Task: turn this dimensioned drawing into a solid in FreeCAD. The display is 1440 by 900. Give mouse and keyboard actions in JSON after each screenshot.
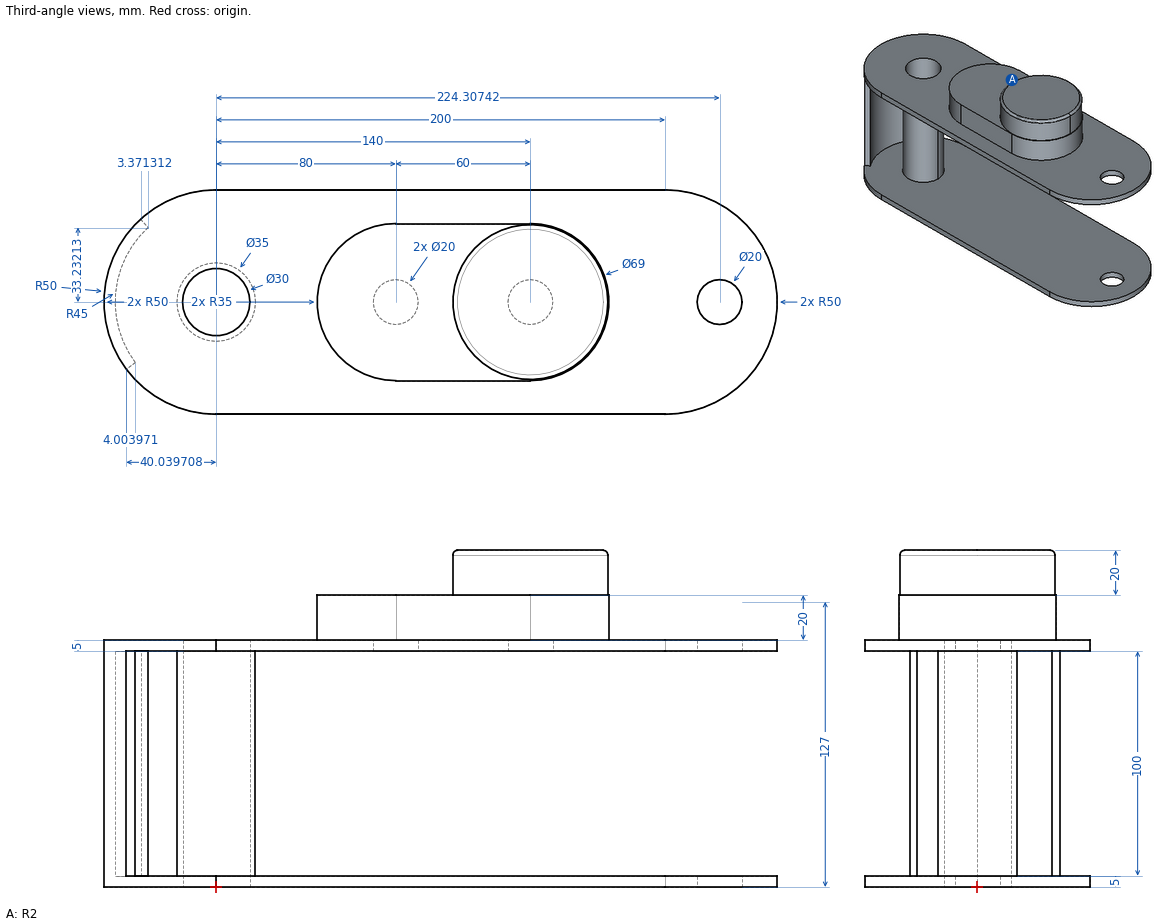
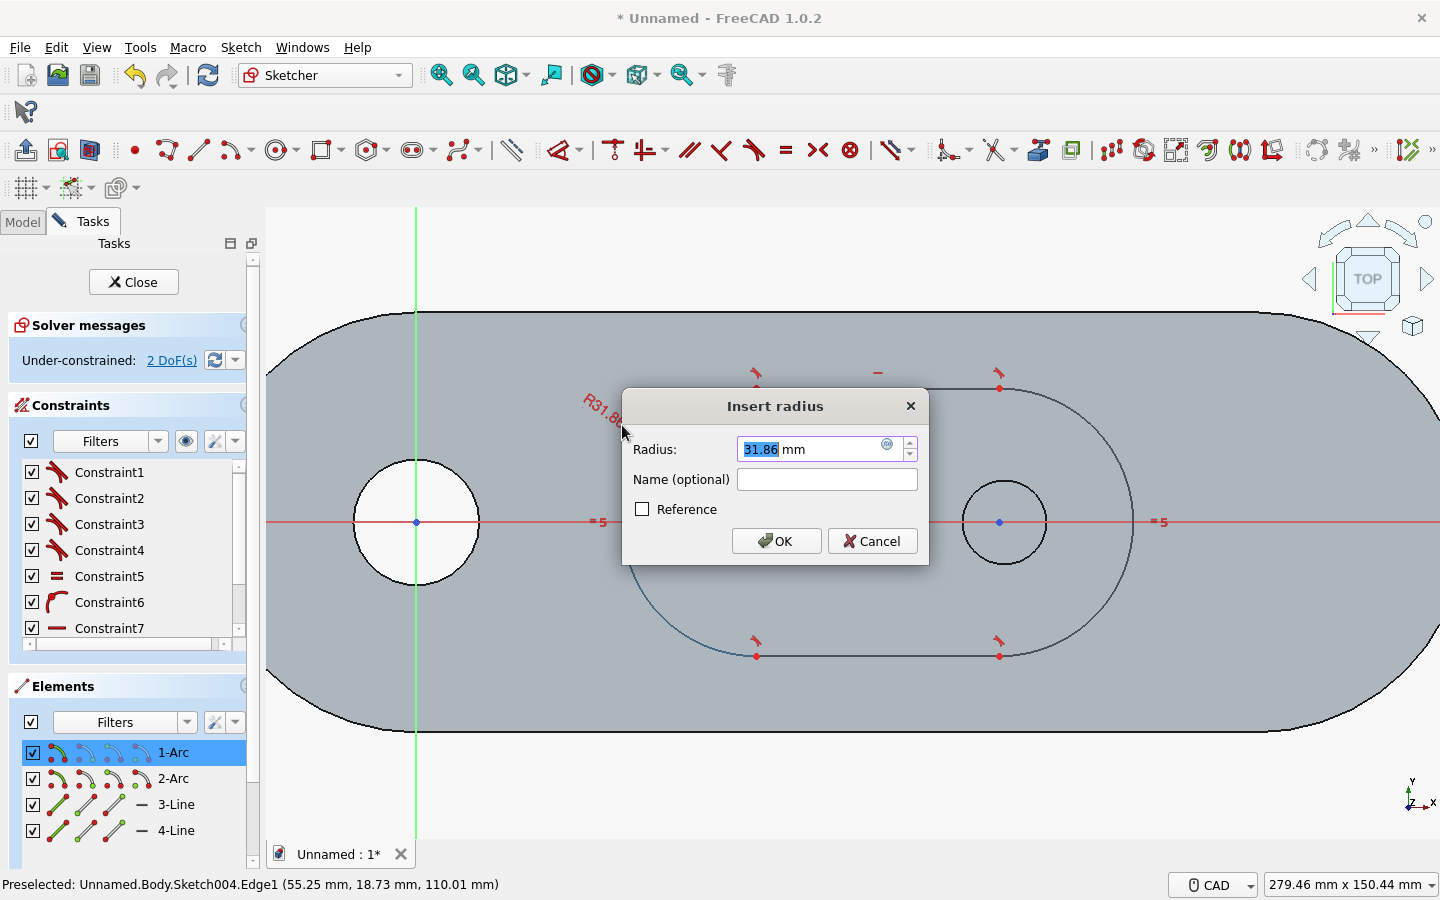
{"action": "type", "text": "35"}
{"action": "key", "text": "Return"}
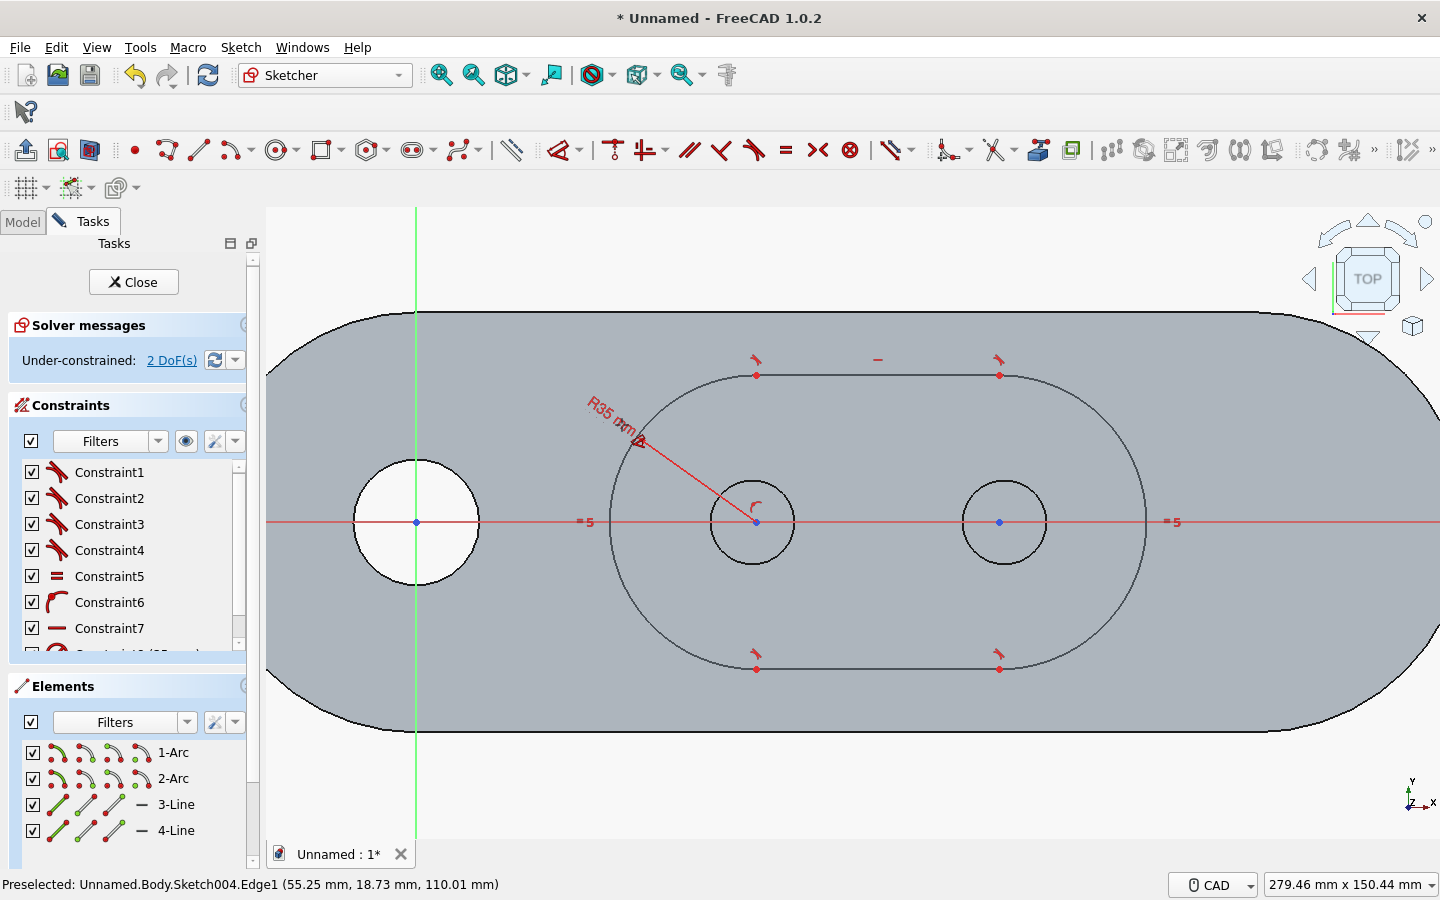
{"action": "left_click", "coordinate": [830, 375]}
{"action": "left_click", "coordinate": [878, 341]}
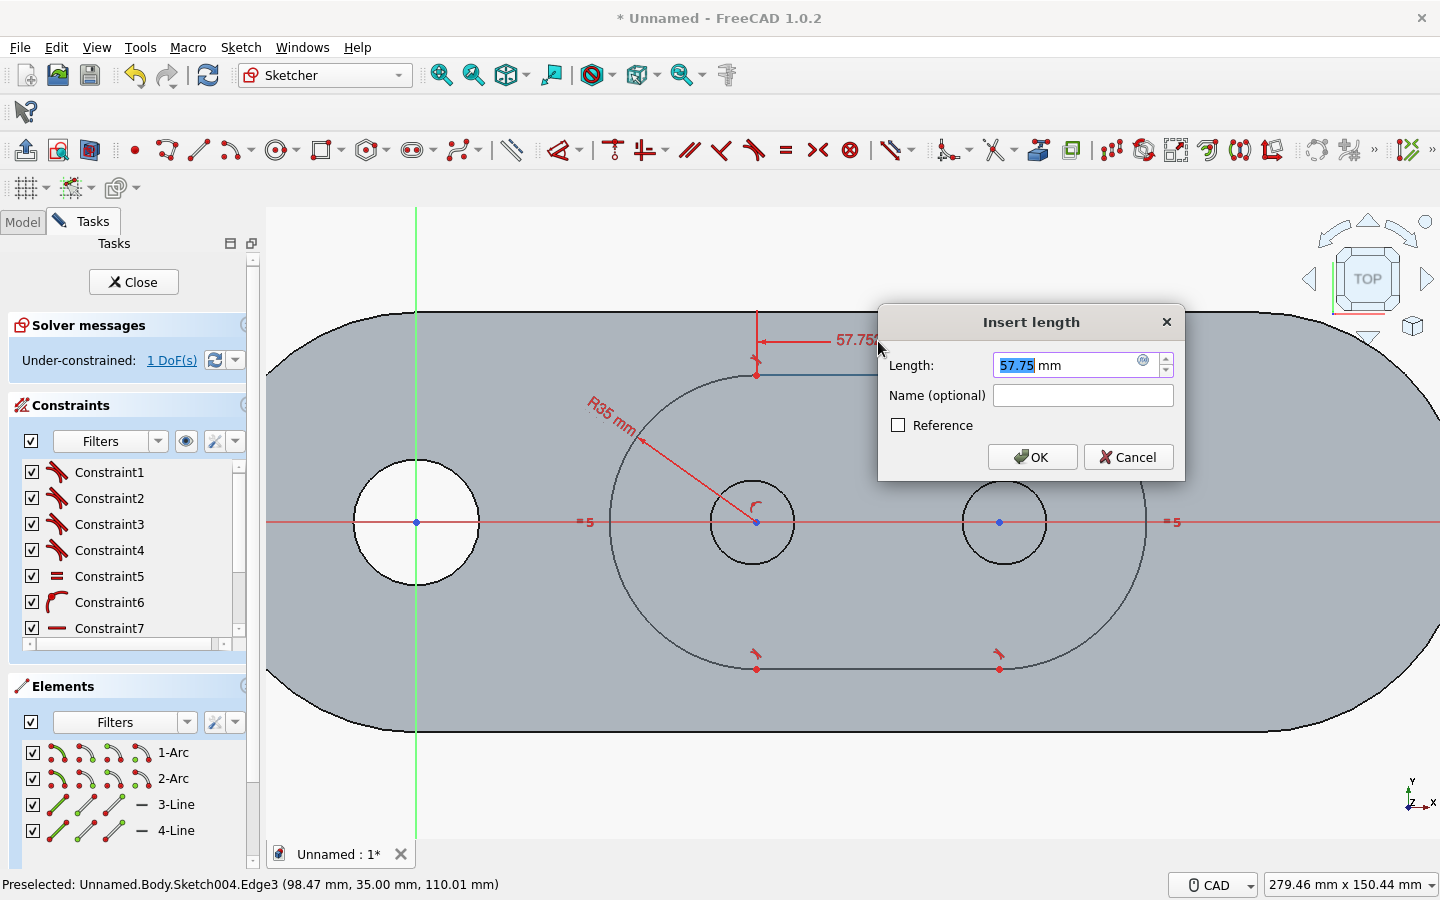
{"action": "type", "text": "60"}
{"action": "key", "text": "Return"}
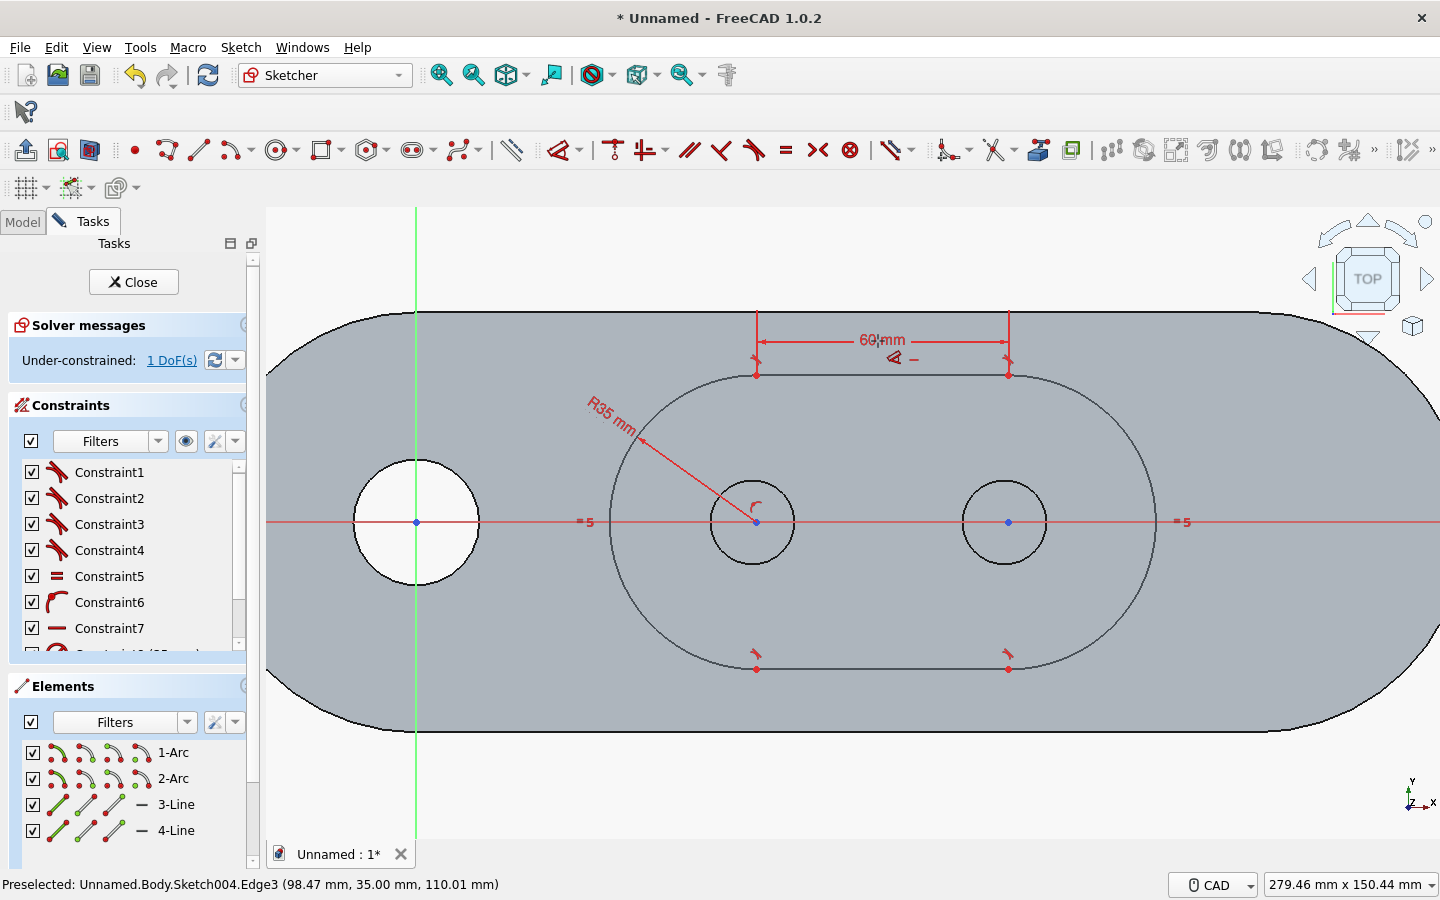
{"action": "left_click", "coordinate": [757, 375]}
{"action": "left_click", "coordinate": [587, 341]}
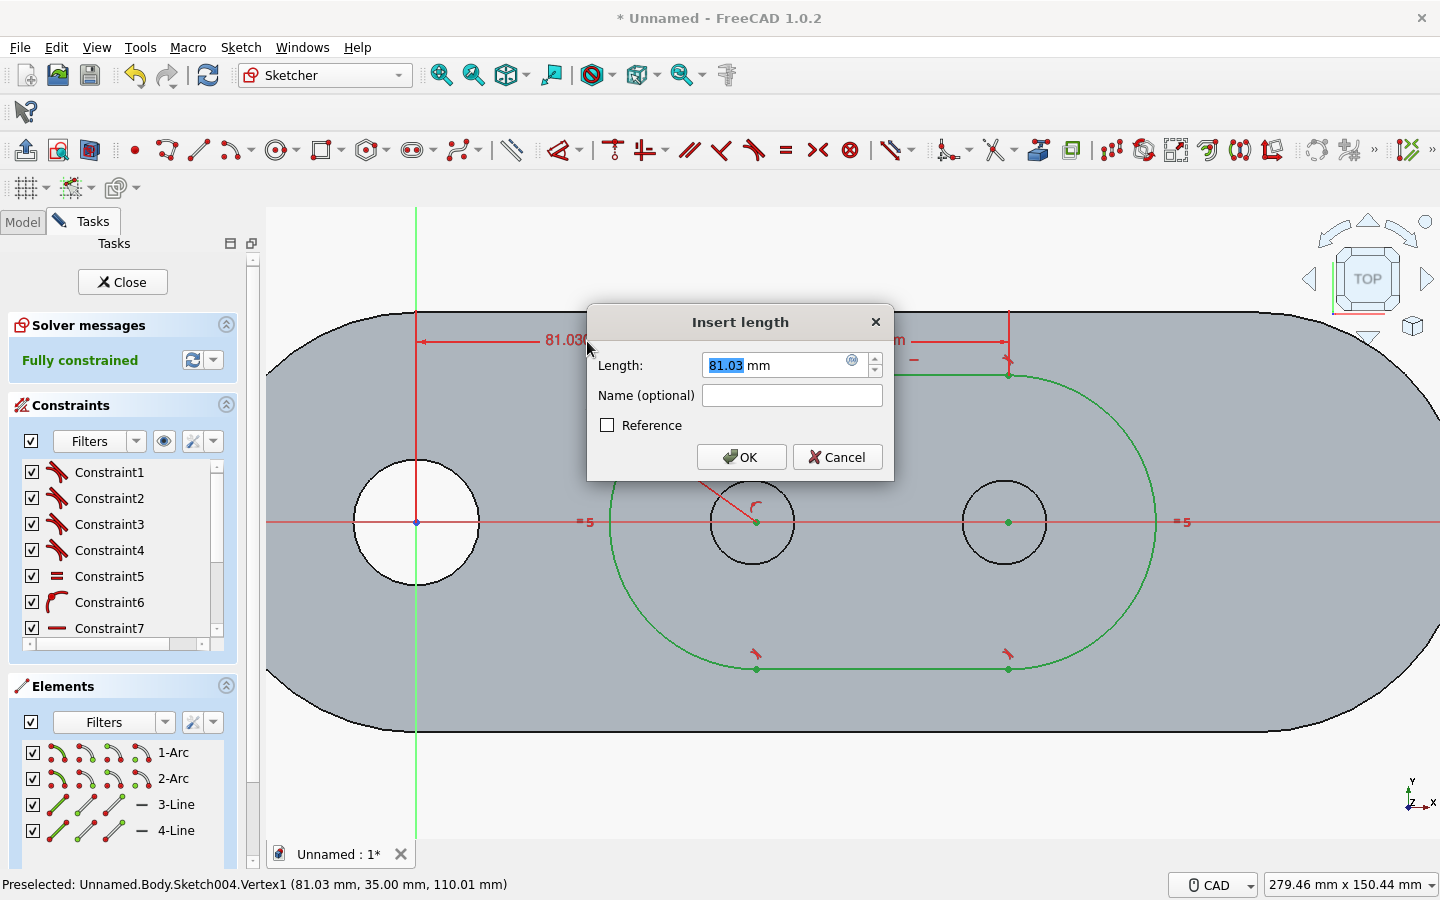
{"action": "type", "text": "80"}
{"action": "key", "text": "Return"}
{"action": "key", "text": "Escape"}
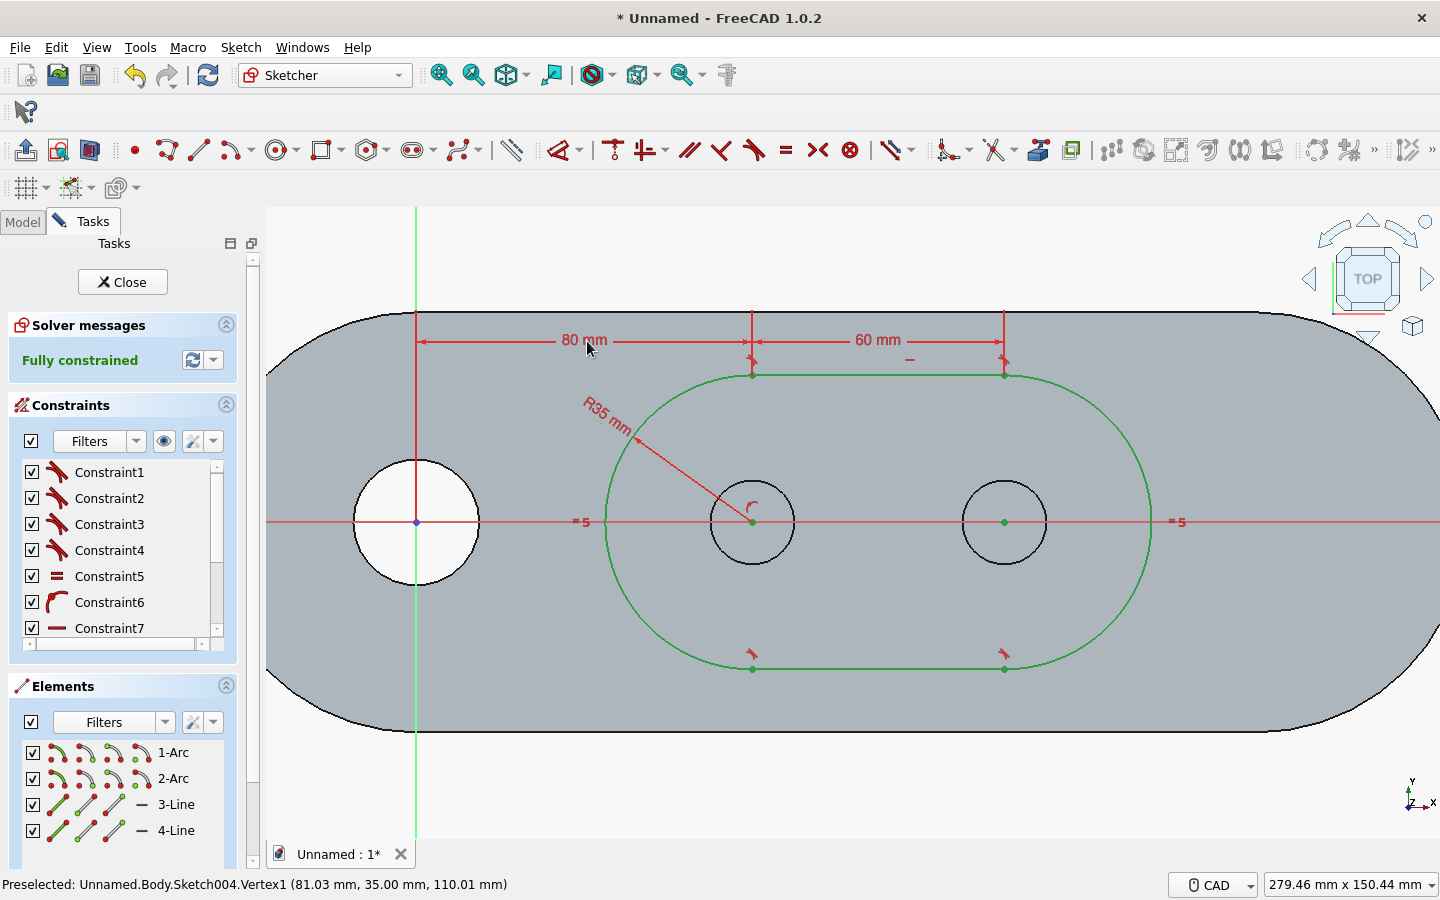
{"action": "left_click", "coordinate": [123, 282]}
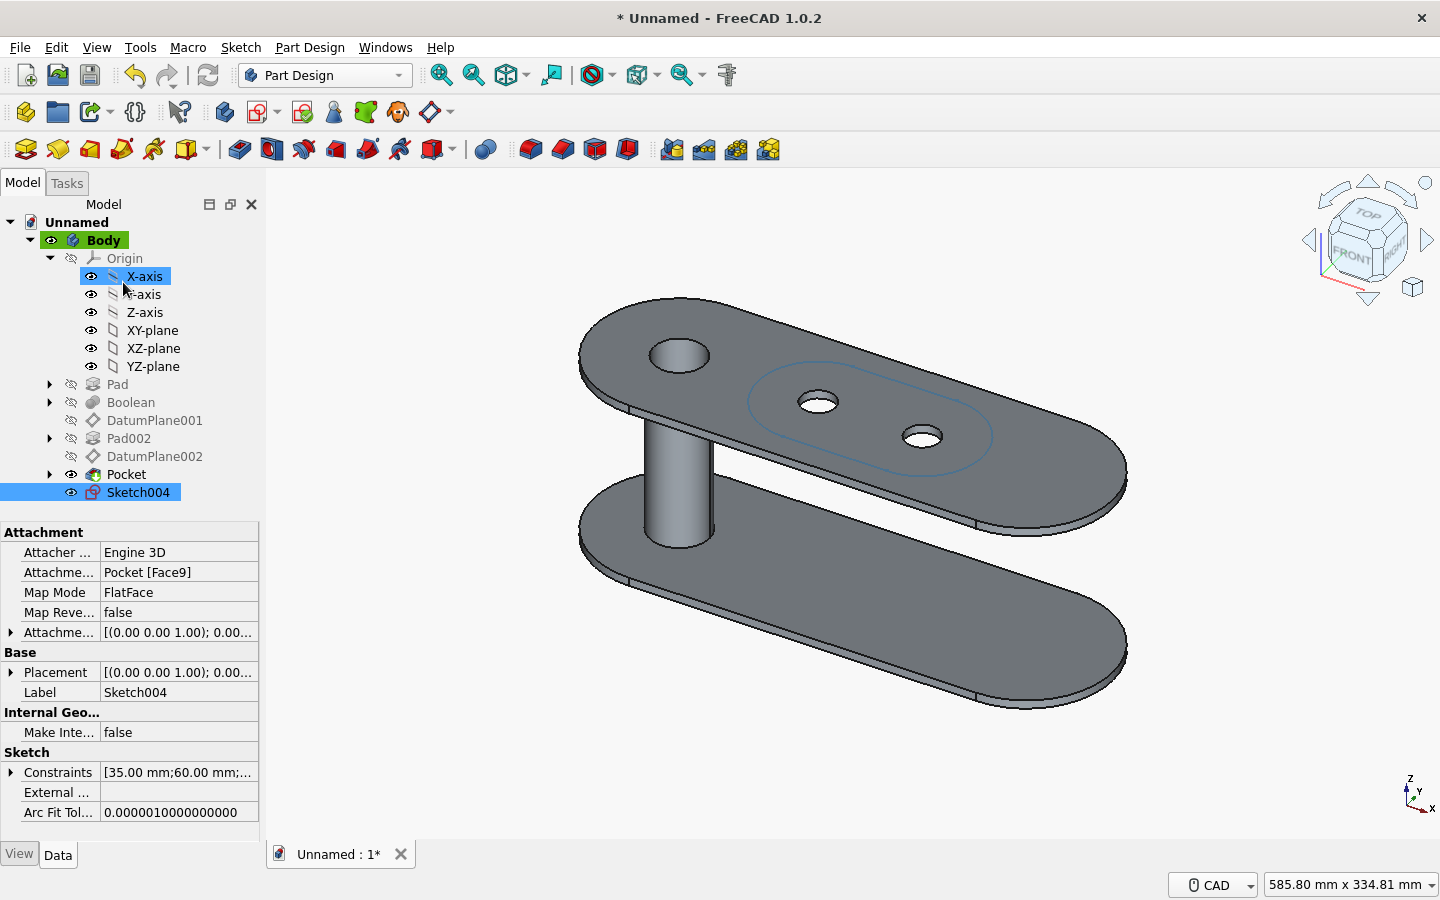
{"action": "left_click", "coordinate": [26, 150]}